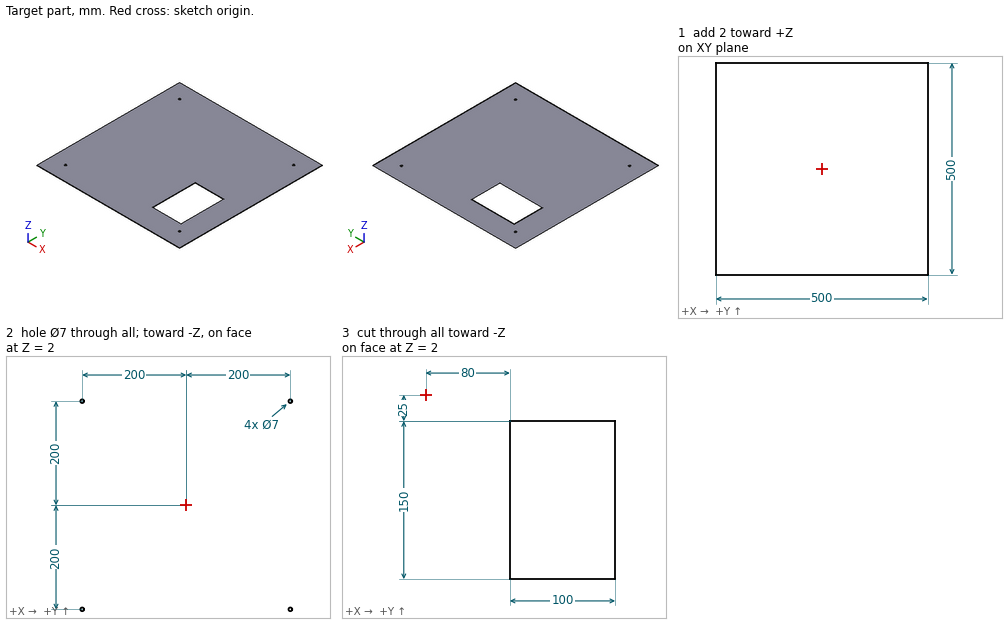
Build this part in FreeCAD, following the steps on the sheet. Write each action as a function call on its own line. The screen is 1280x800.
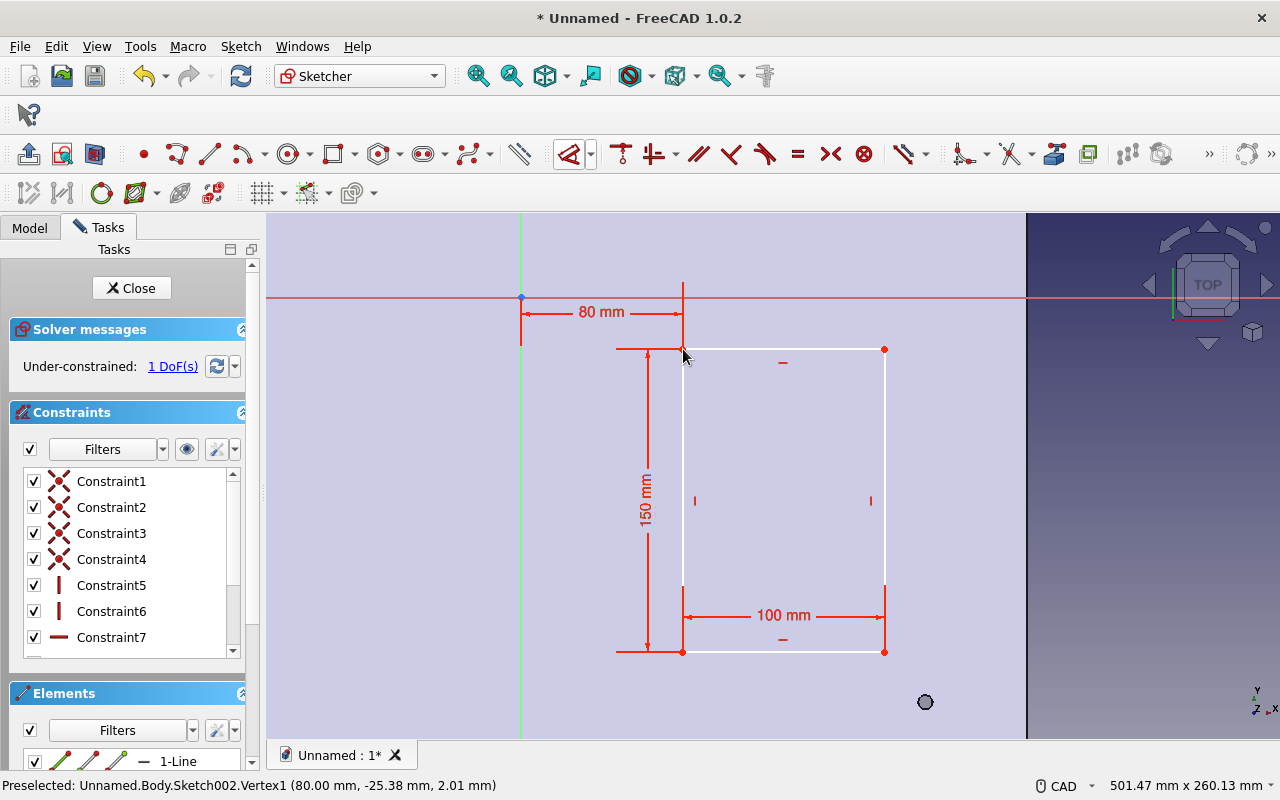
click(683, 349)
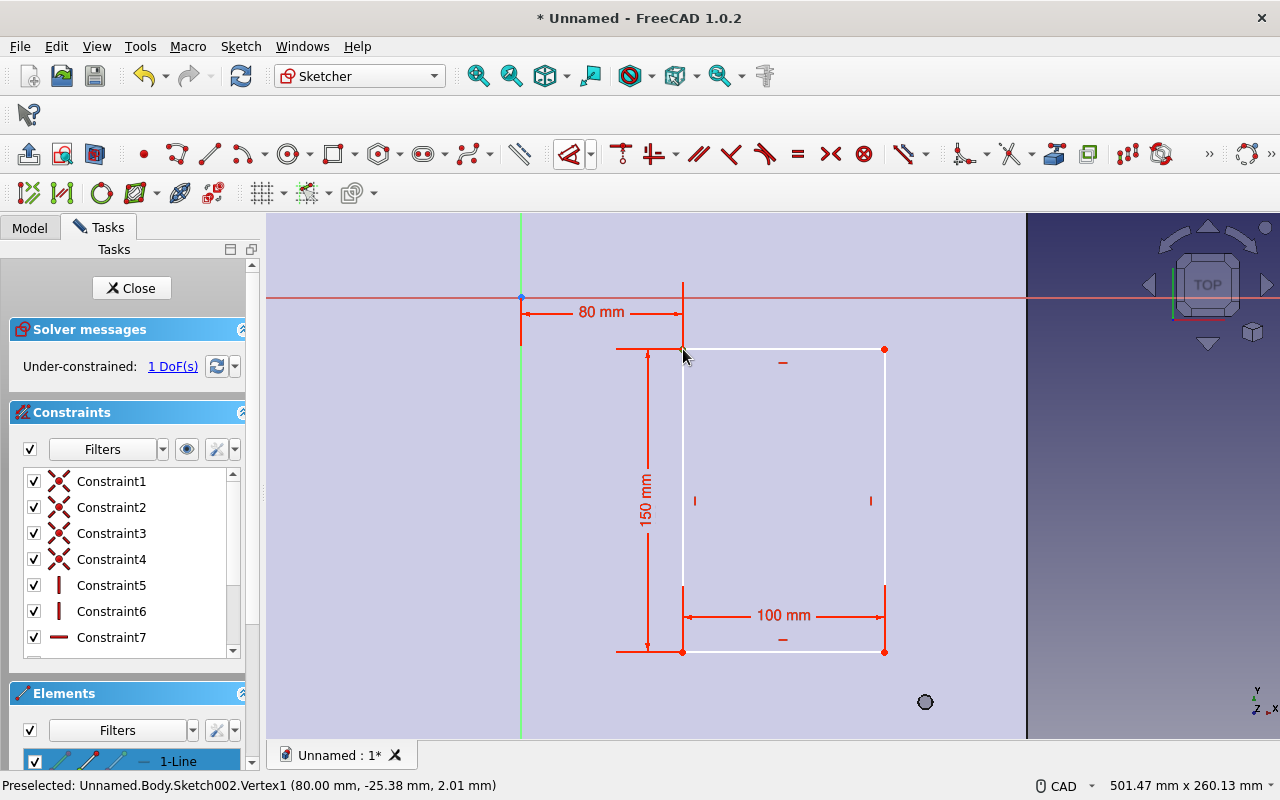
key(i)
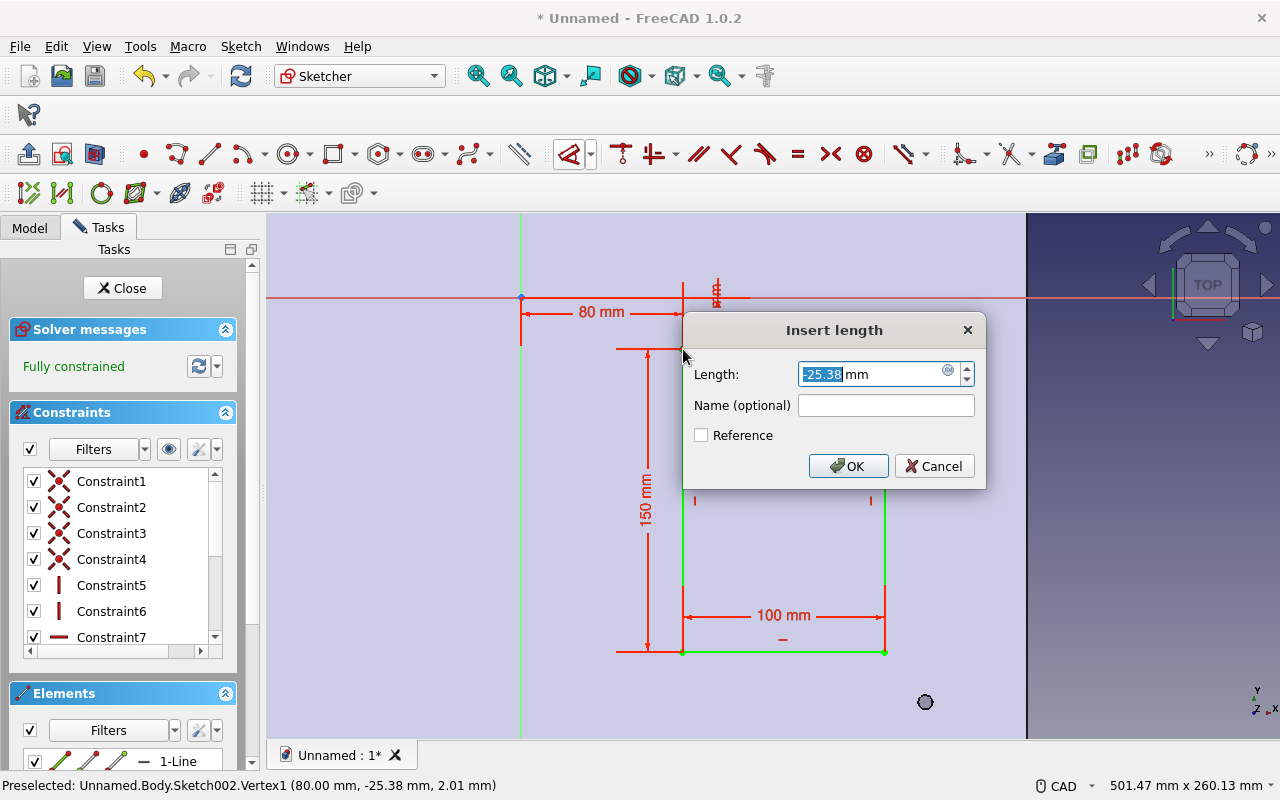
text(-25)
key(Return)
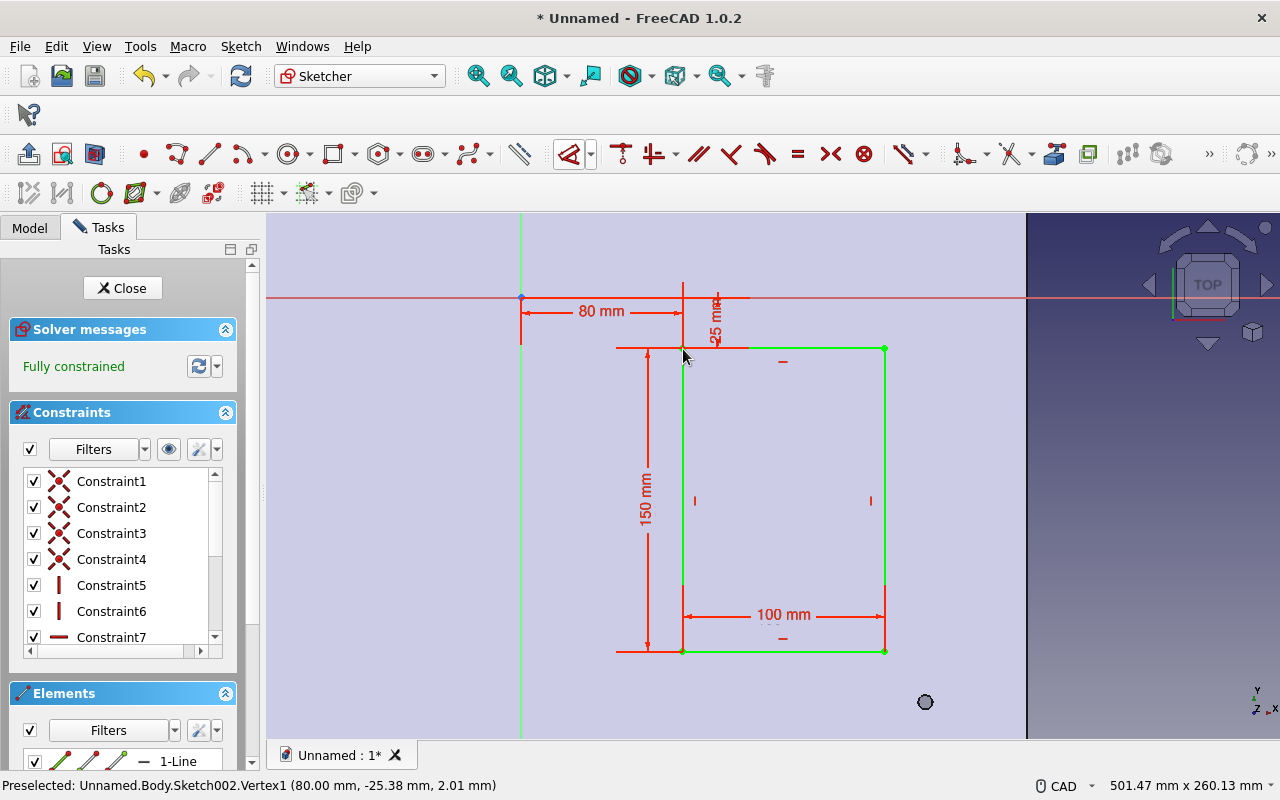
click(123, 288)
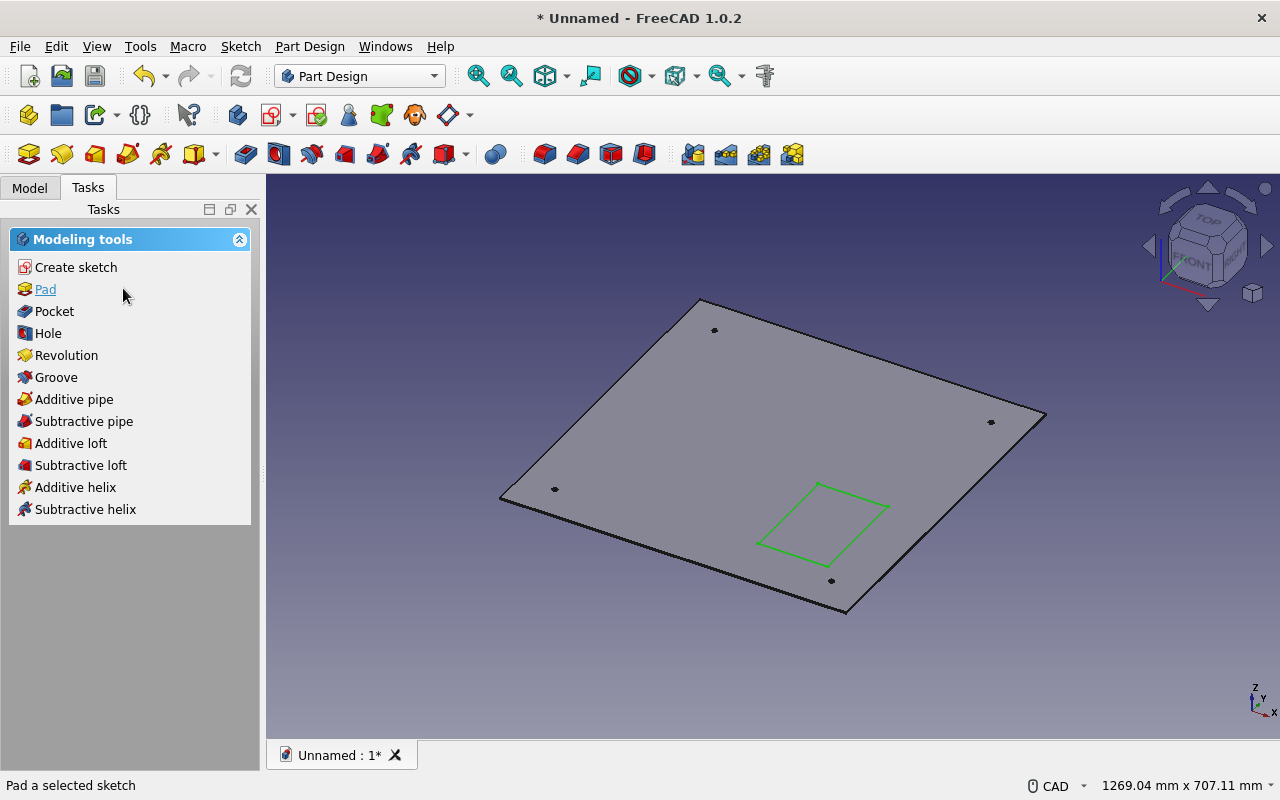
click(246, 154)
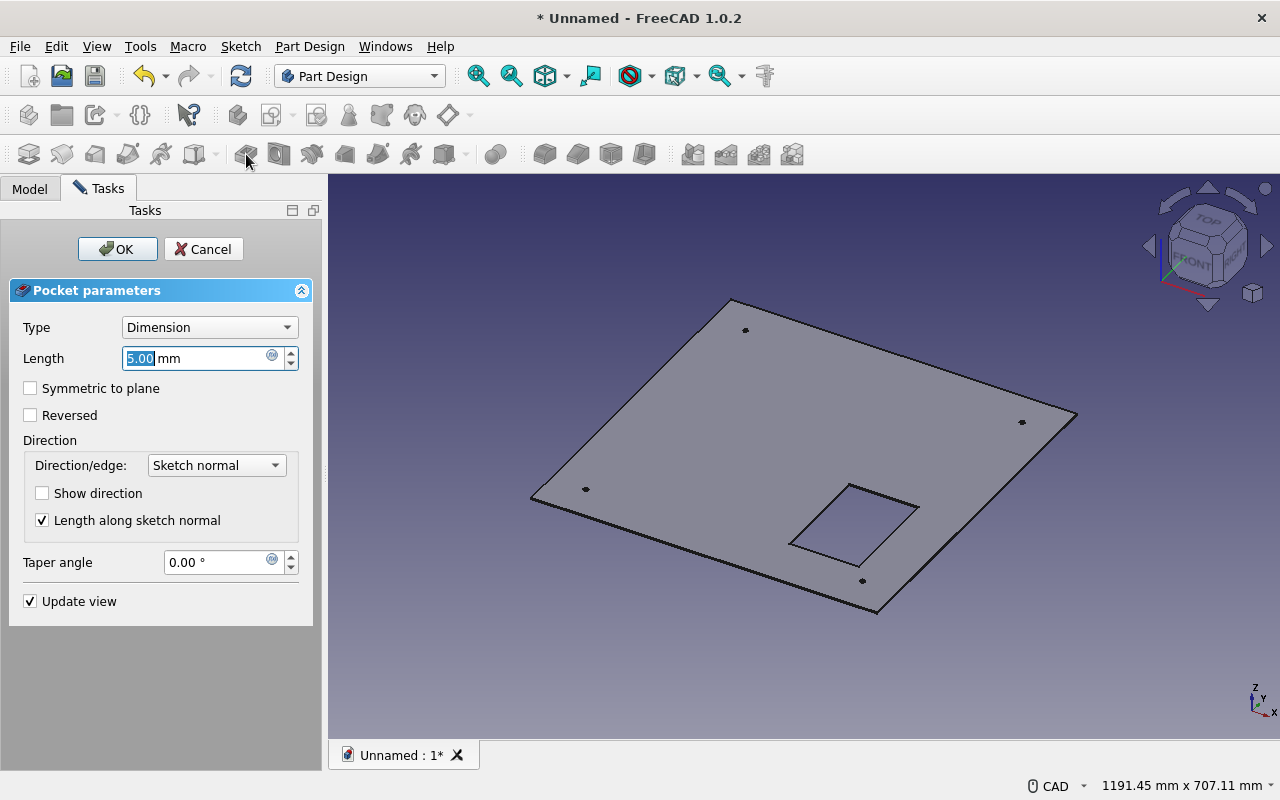
click(210, 328)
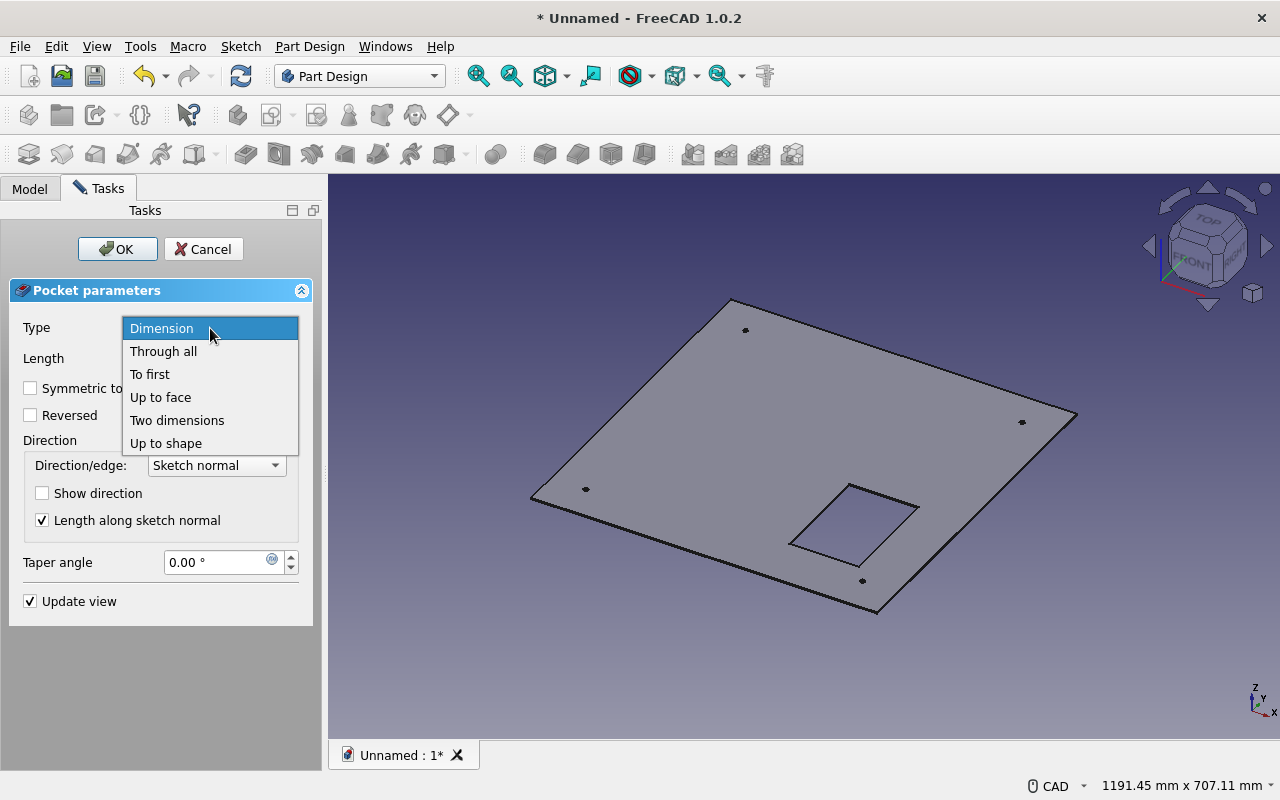
click(208, 352)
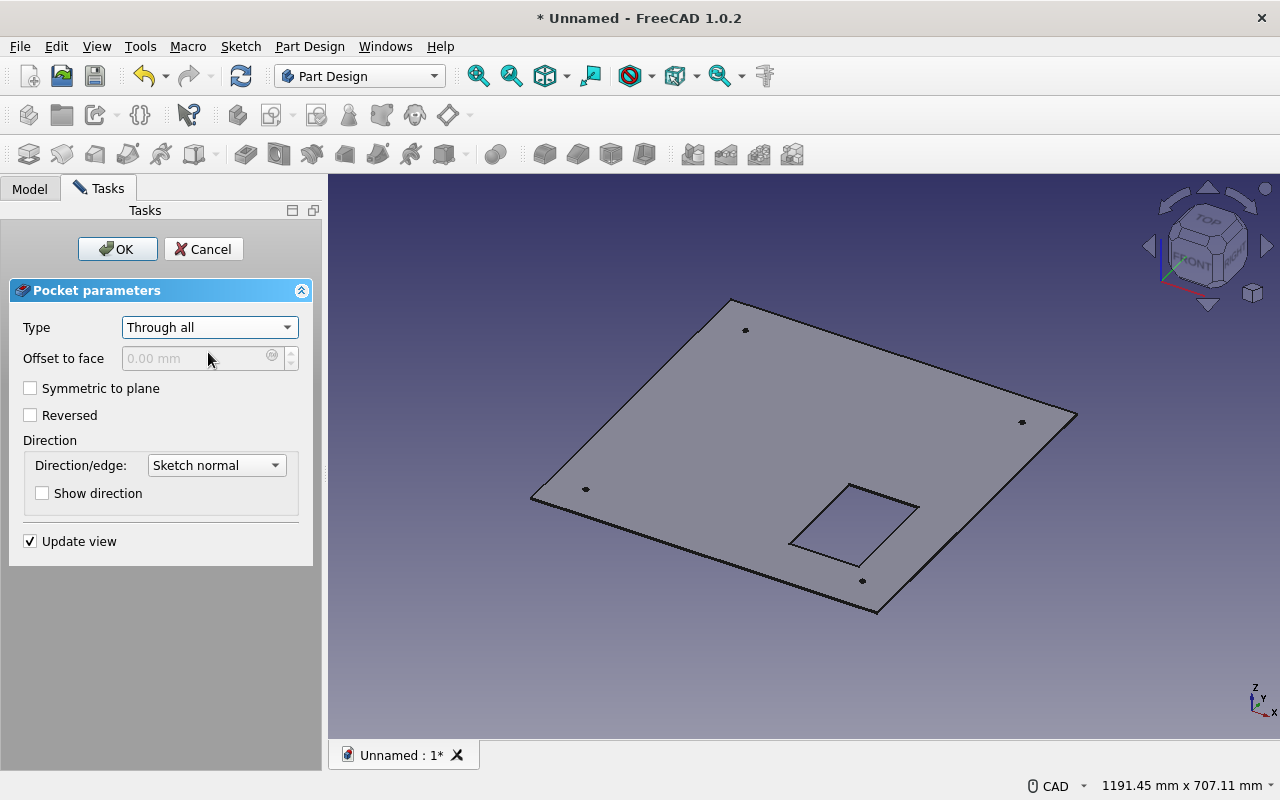
click(118, 249)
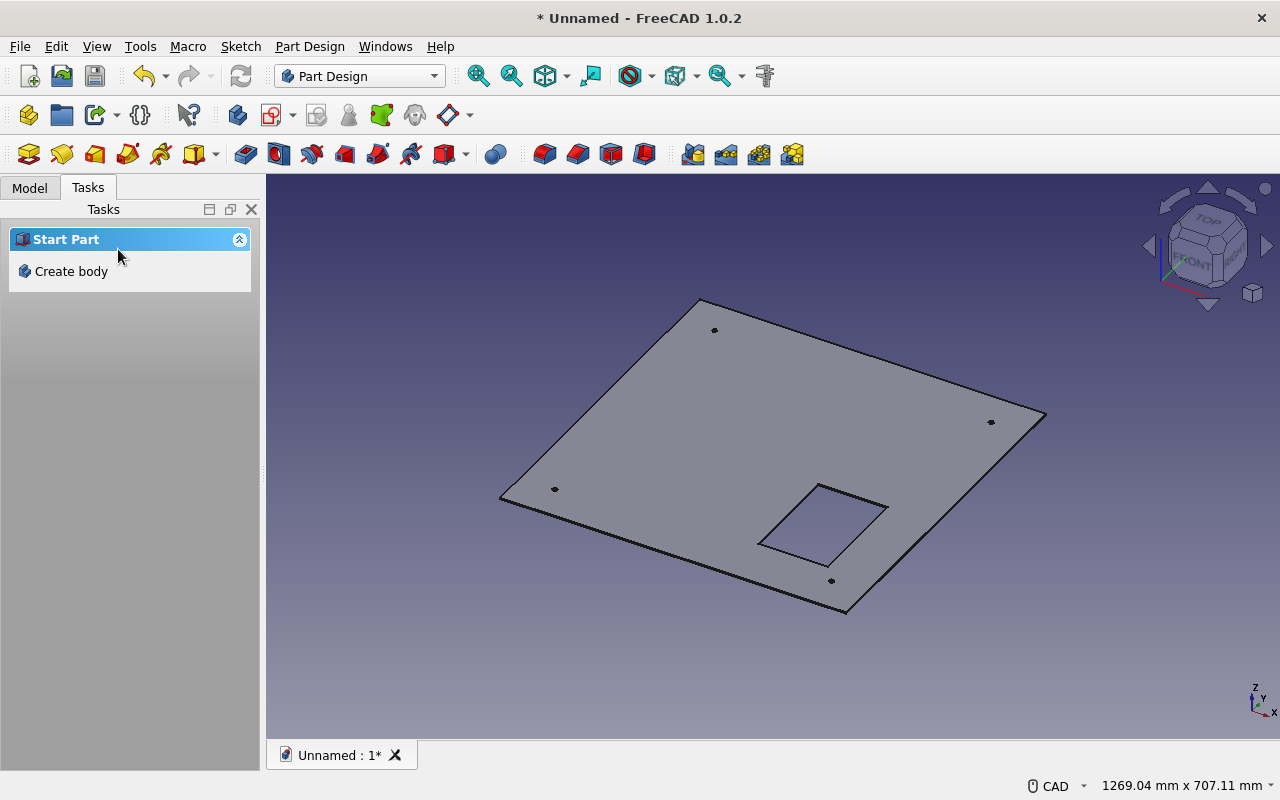
key(0)